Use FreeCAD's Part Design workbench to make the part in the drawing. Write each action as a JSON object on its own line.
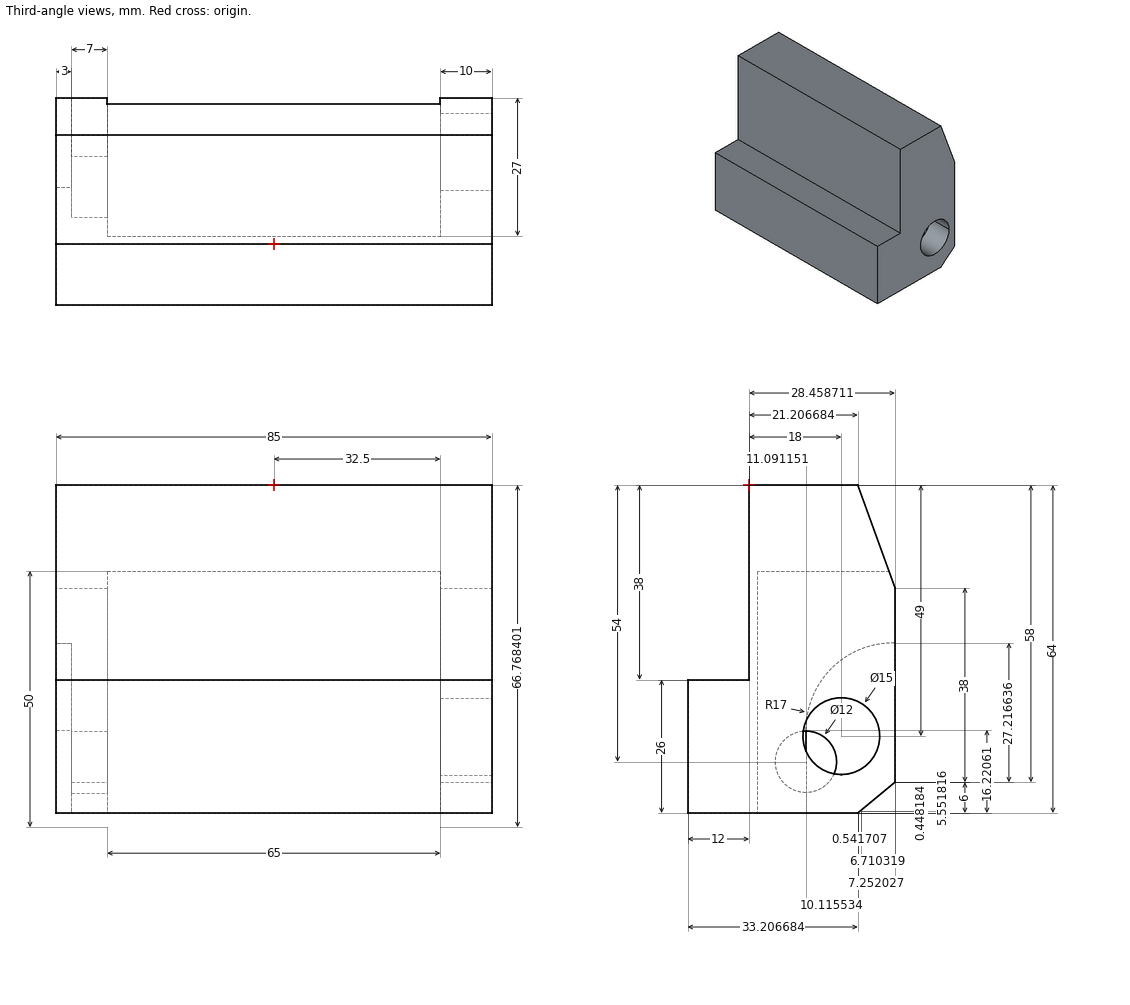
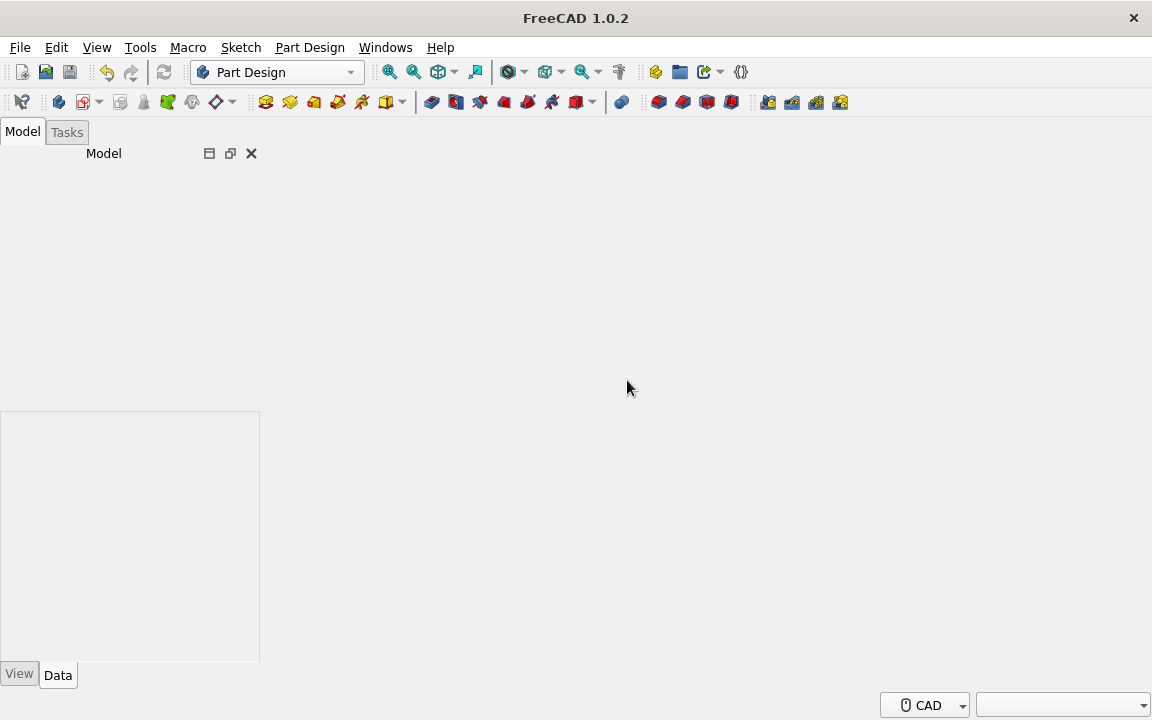
{"action": "left_click", "coordinate": [22, 72]}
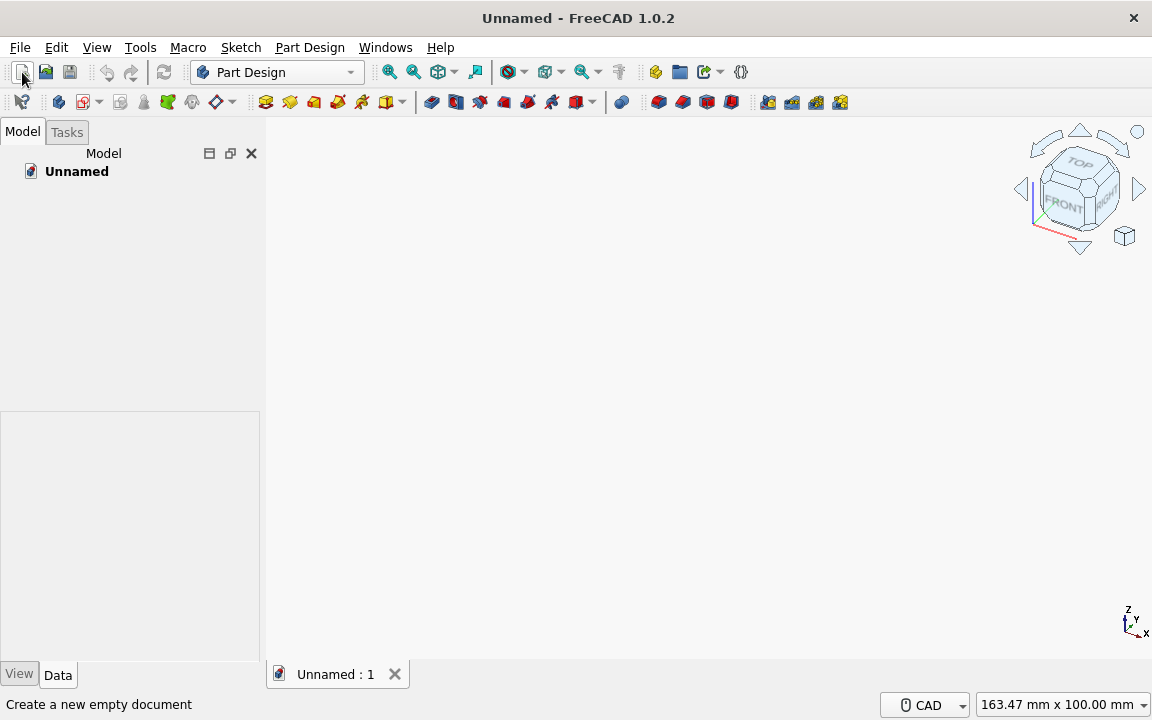
{"action": "left_click", "coordinate": [84, 102]}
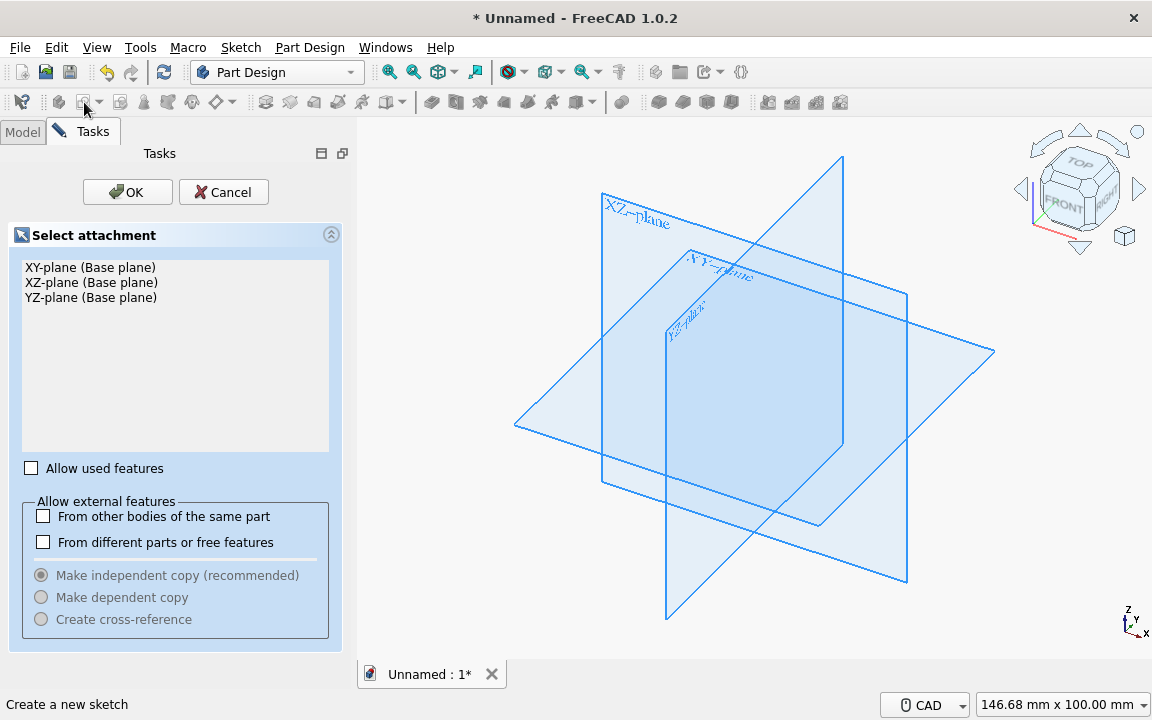
{"action": "left_click", "coordinate": [82, 298]}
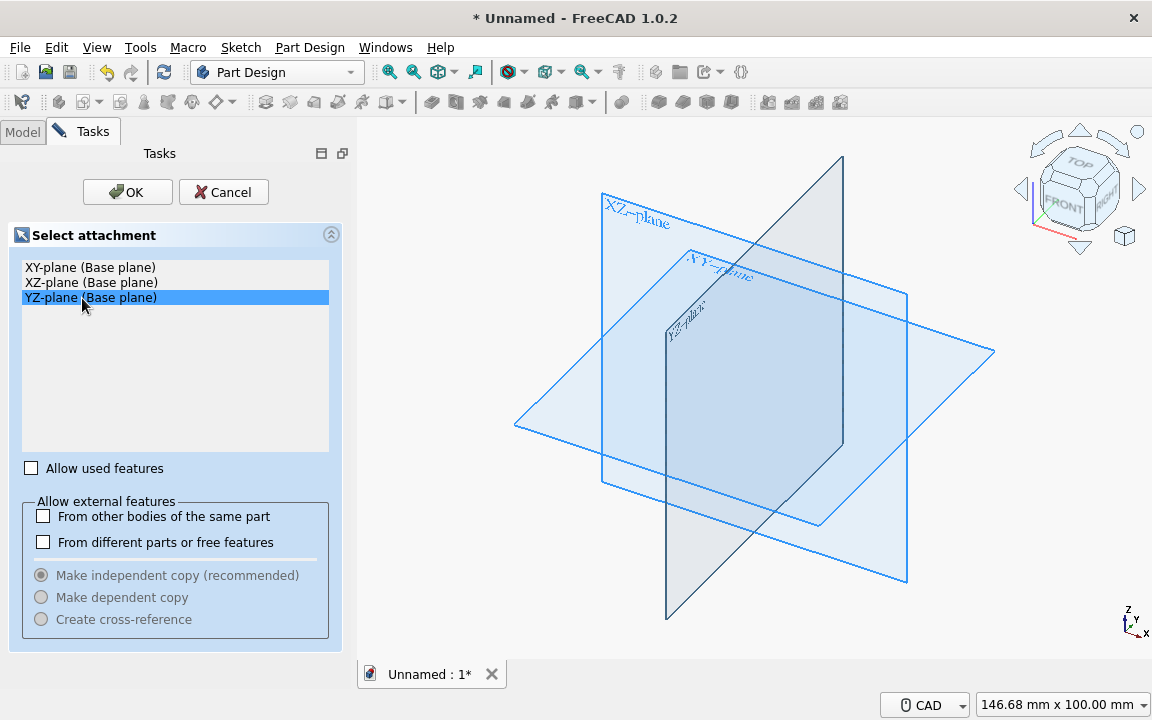
{"action": "left_click", "coordinate": [128, 192]}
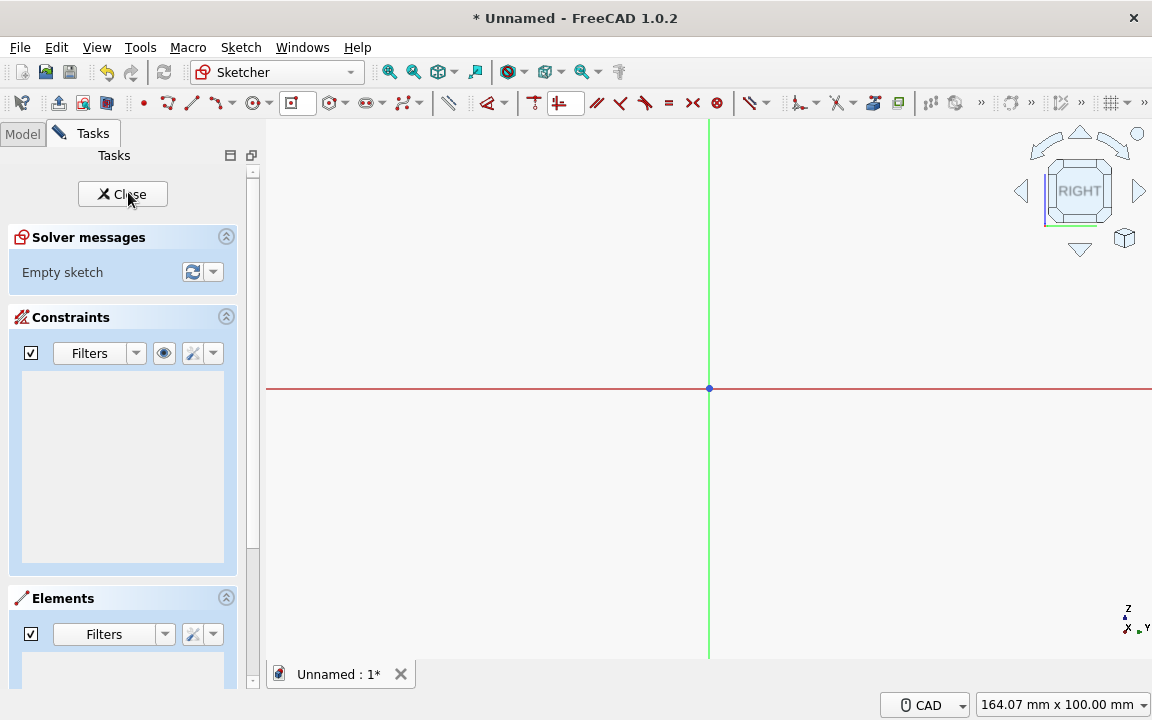
{"action": "scroll", "coordinate": [411, 147], "scroll_direction": "down", "scroll_amount": 2}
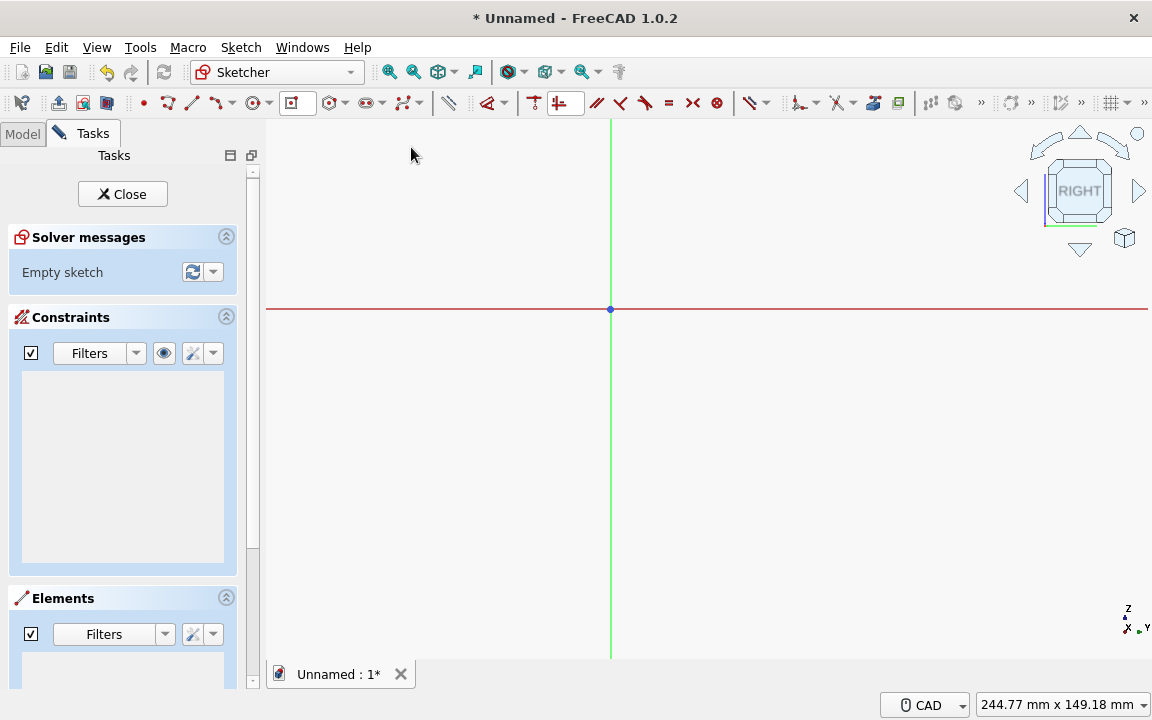
{"action": "scroll", "coordinate": [641, 498], "scroll_direction": "up", "scroll_amount": 2}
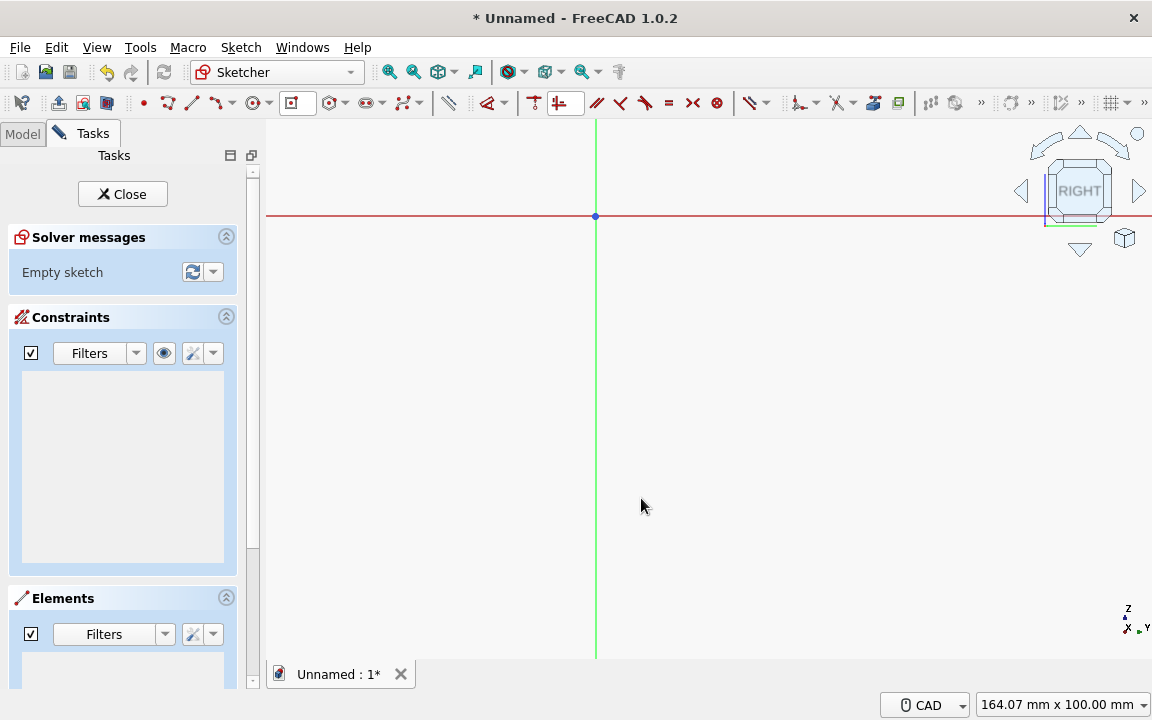
{"action": "left_click", "coordinate": [168, 104]}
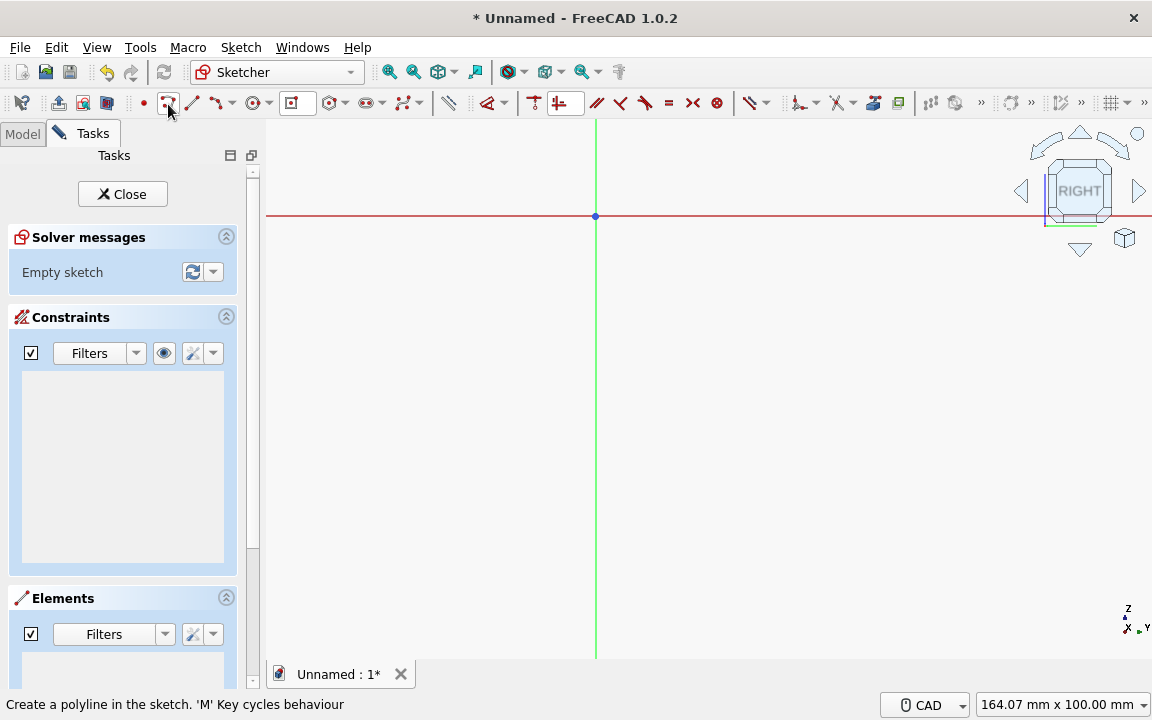
{"action": "left_click", "coordinate": [596, 216]}
{"action": "left_click", "coordinate": [605, 421]}
{"action": "left_click", "coordinate": [531, 421]}
{"action": "left_click", "coordinate": [531, 562]}
{"action": "left_click", "coordinate": [710, 562]}
{"action": "left_click", "coordinate": [749, 529]}
{"action": "left_click", "coordinate": [749, 324]}
{"action": "left_click", "coordinate": [710, 225]}
{"action": "left_click", "coordinate": [596, 216]}
{"action": "key", "text": "Escape"}
{"action": "key", "text": "Escape"}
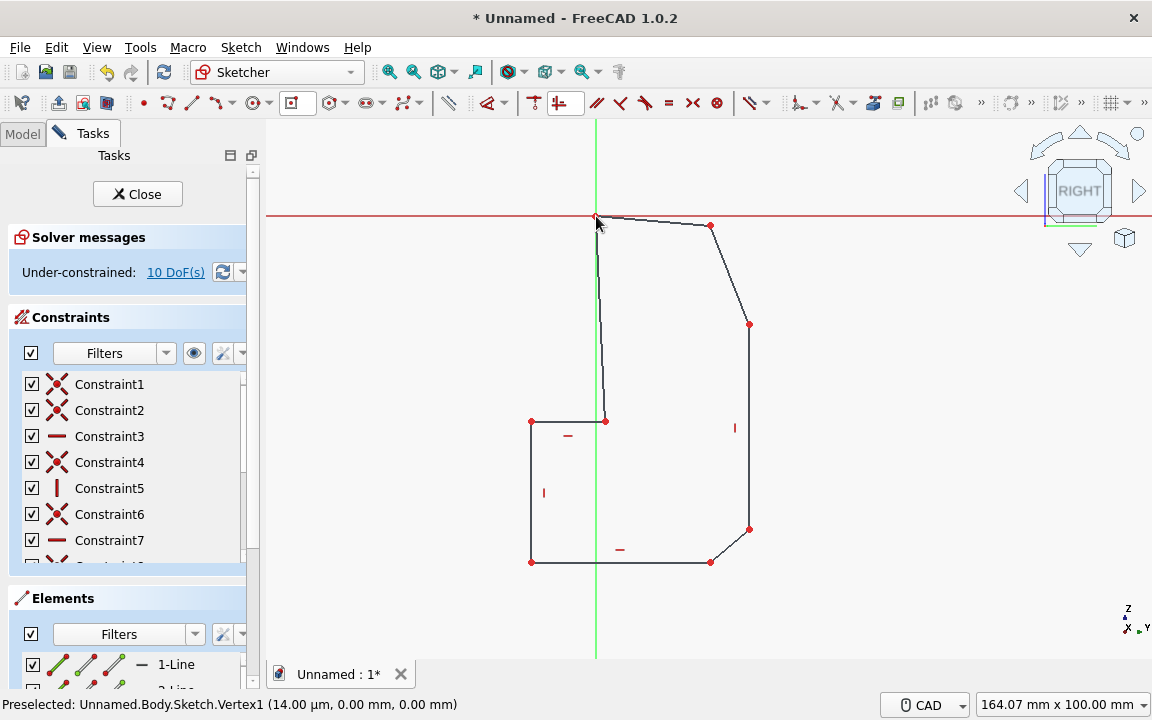
{"action": "left_click", "coordinate": [599, 278]}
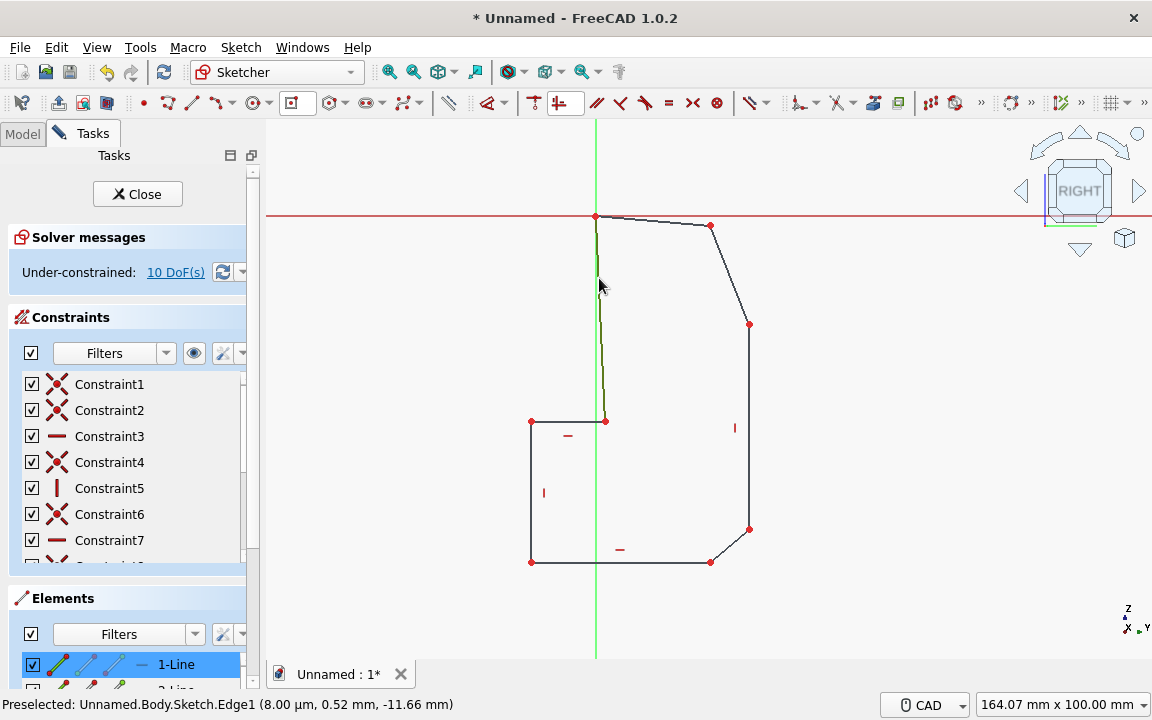
{"action": "left_click", "coordinate": [578, 104]}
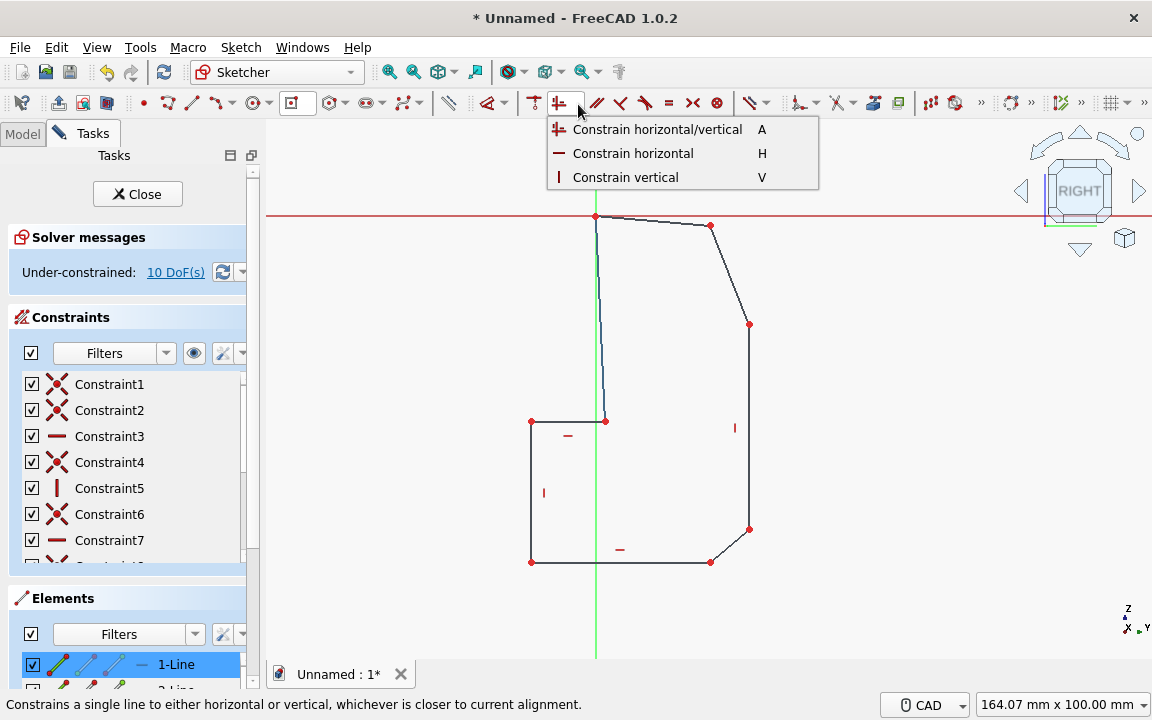
{"action": "left_click", "coordinate": [683, 177]}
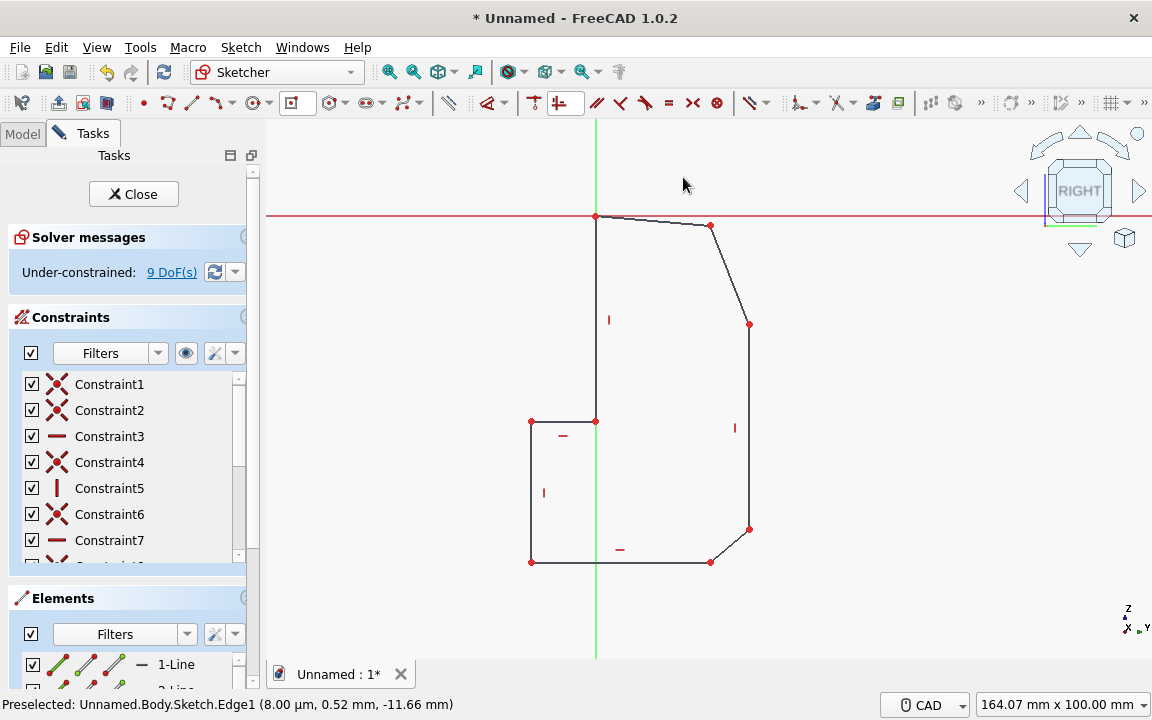
{"action": "left_click", "coordinate": [630, 219]}